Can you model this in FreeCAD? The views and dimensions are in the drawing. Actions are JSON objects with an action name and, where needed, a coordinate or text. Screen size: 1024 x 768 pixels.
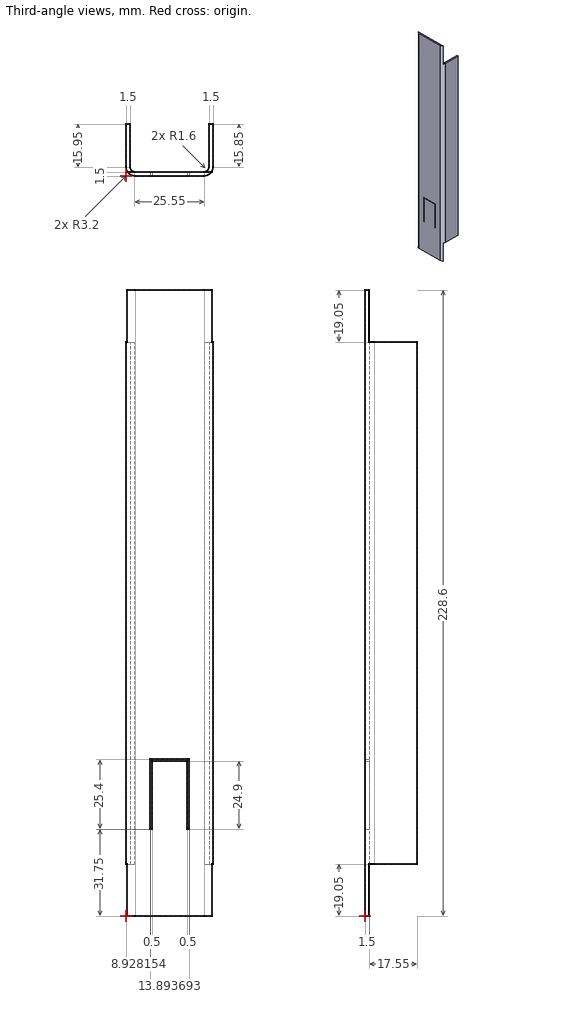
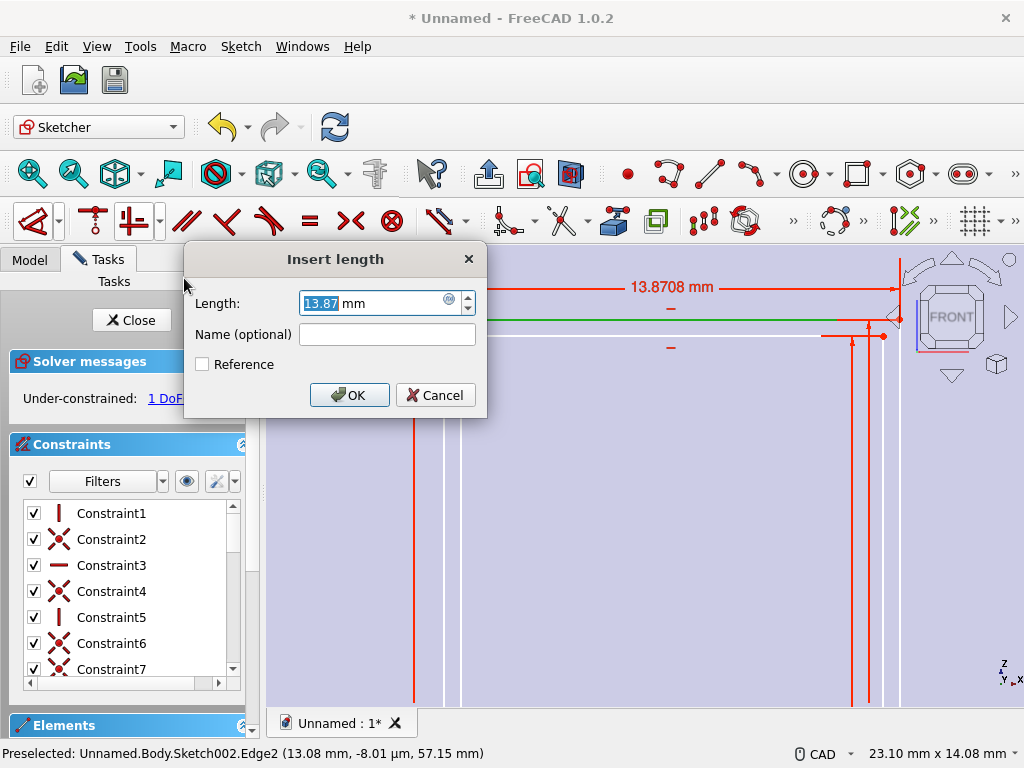
{"action": "type", "text": "13.893693"}
{"action": "key", "text": "Return"}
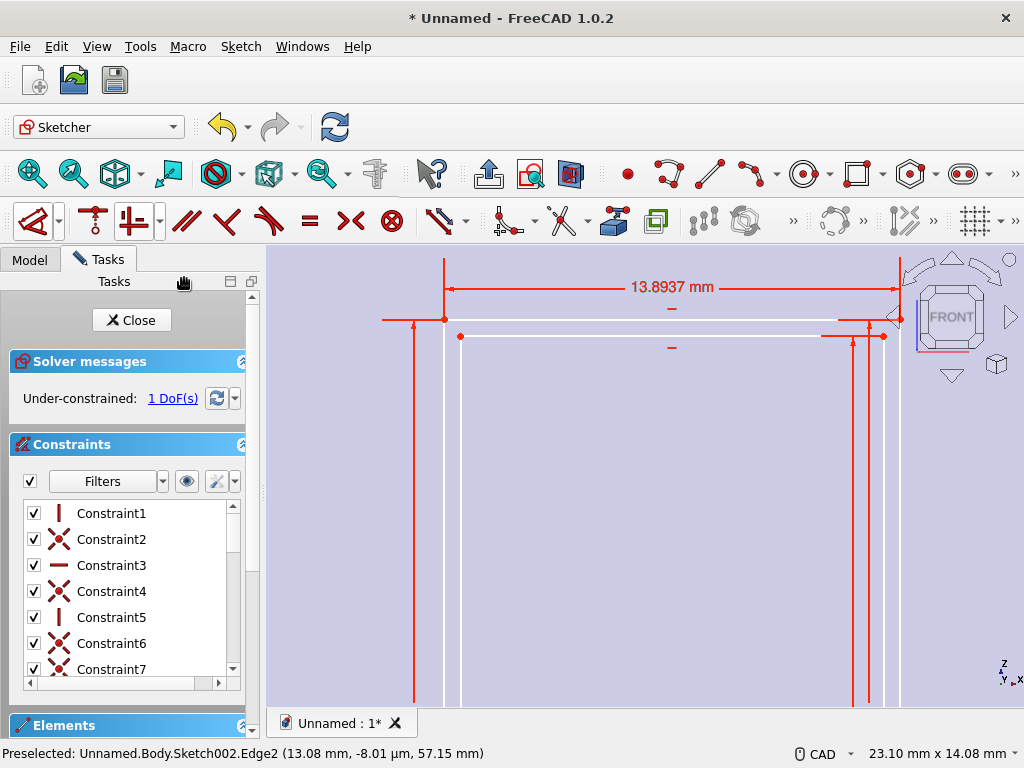
{"action": "scroll", "coordinate": [586, 321], "scroll_direction": "down", "scroll_amount": 9}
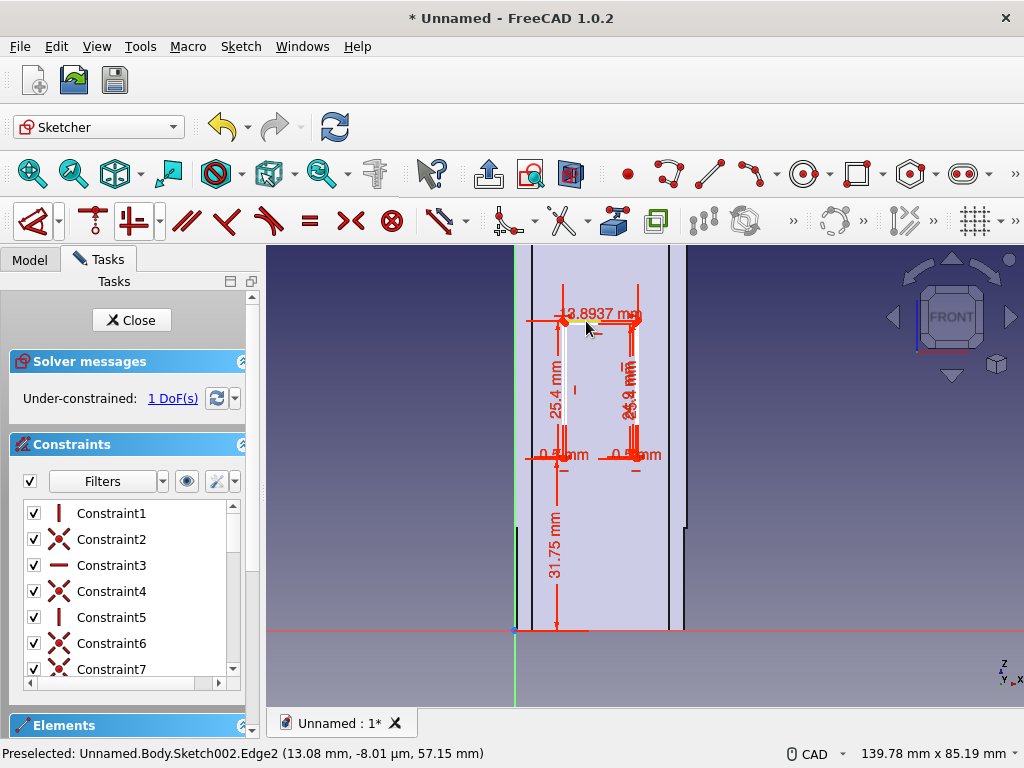
{"action": "scroll", "coordinate": [563, 459], "scroll_direction": "up", "scroll_amount": 8}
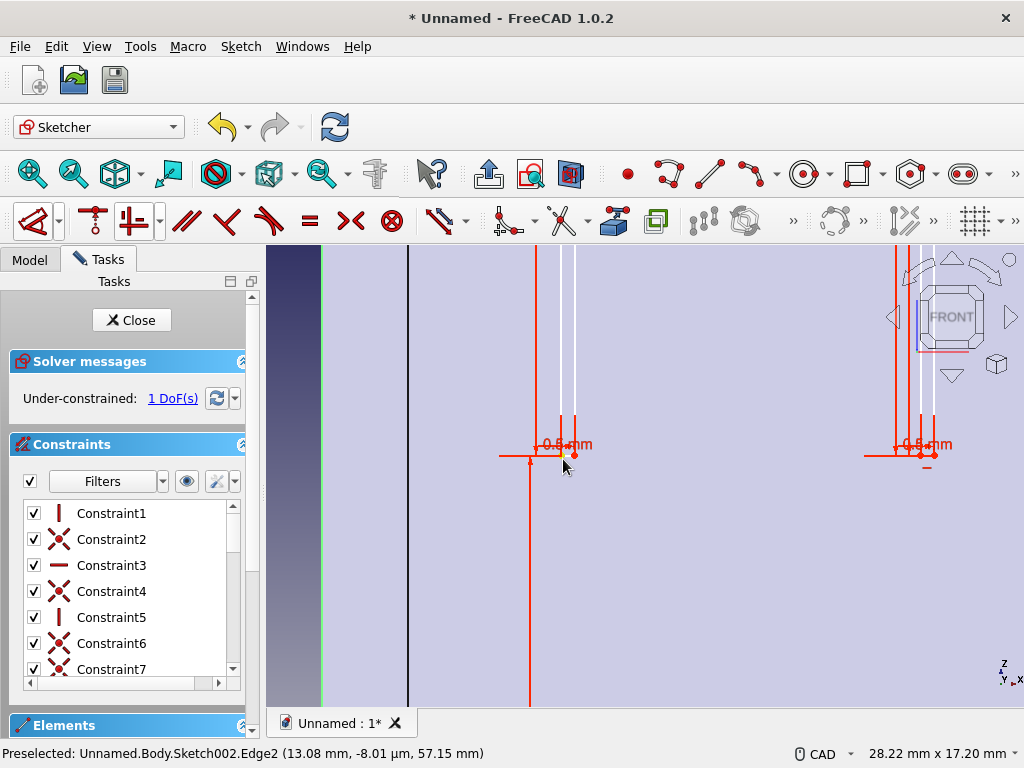
{"action": "left_click", "coordinate": [561, 456]}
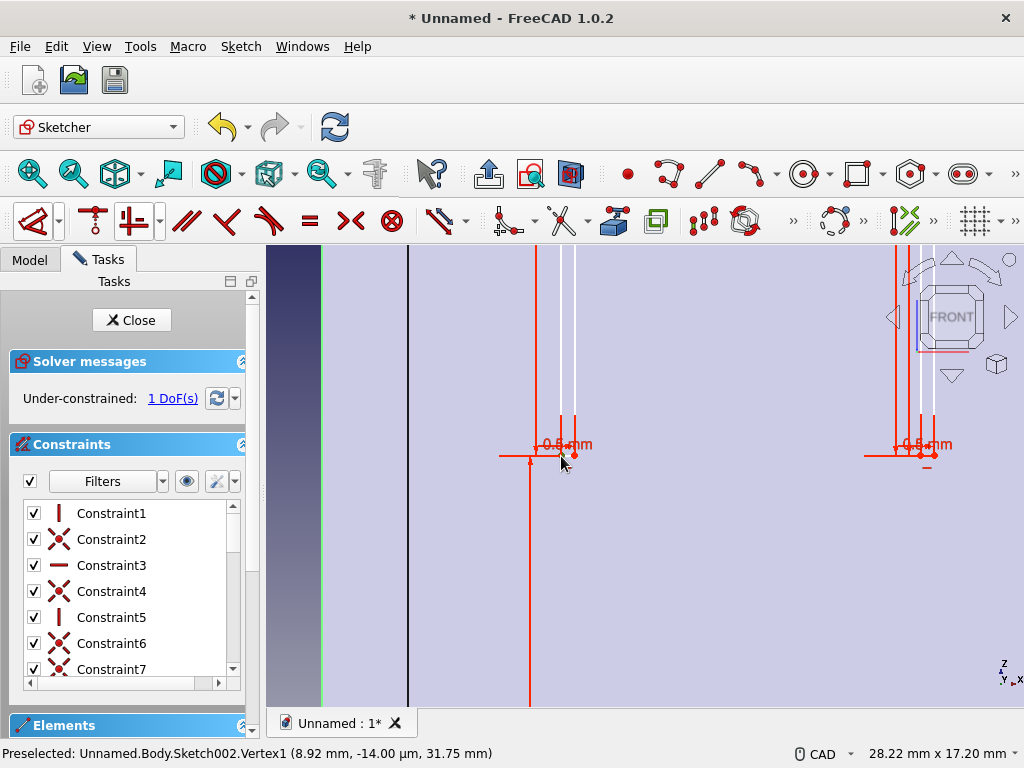
{"action": "left_click", "coordinate": [58, 222]}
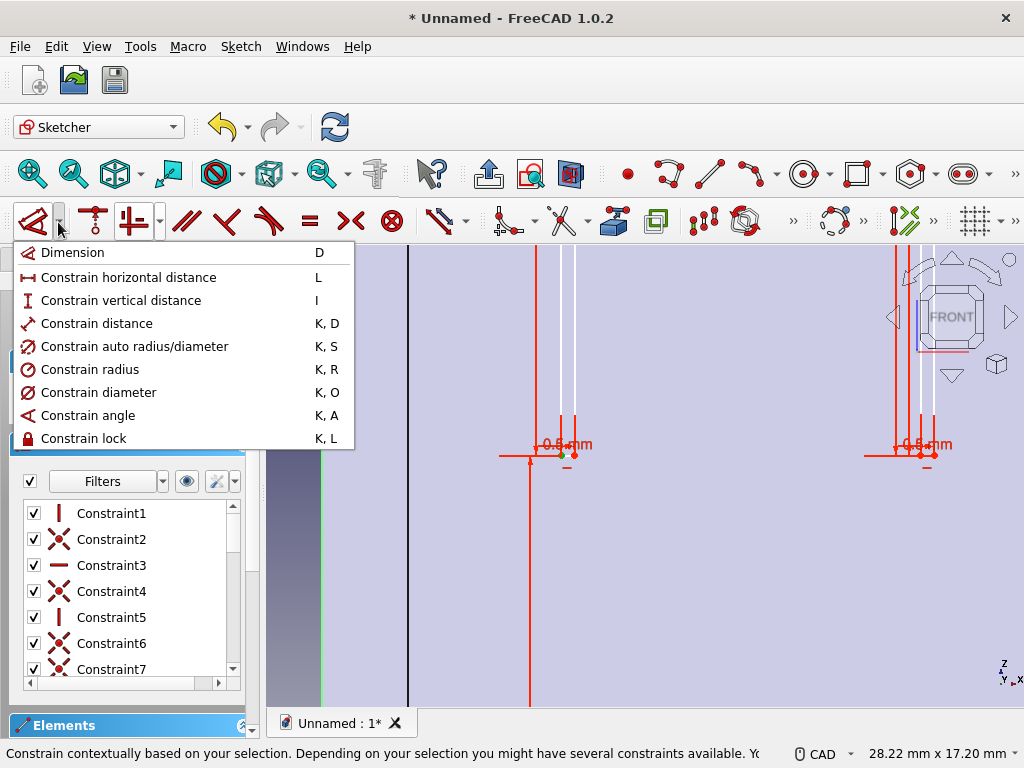
{"action": "left_click", "coordinate": [184, 278]}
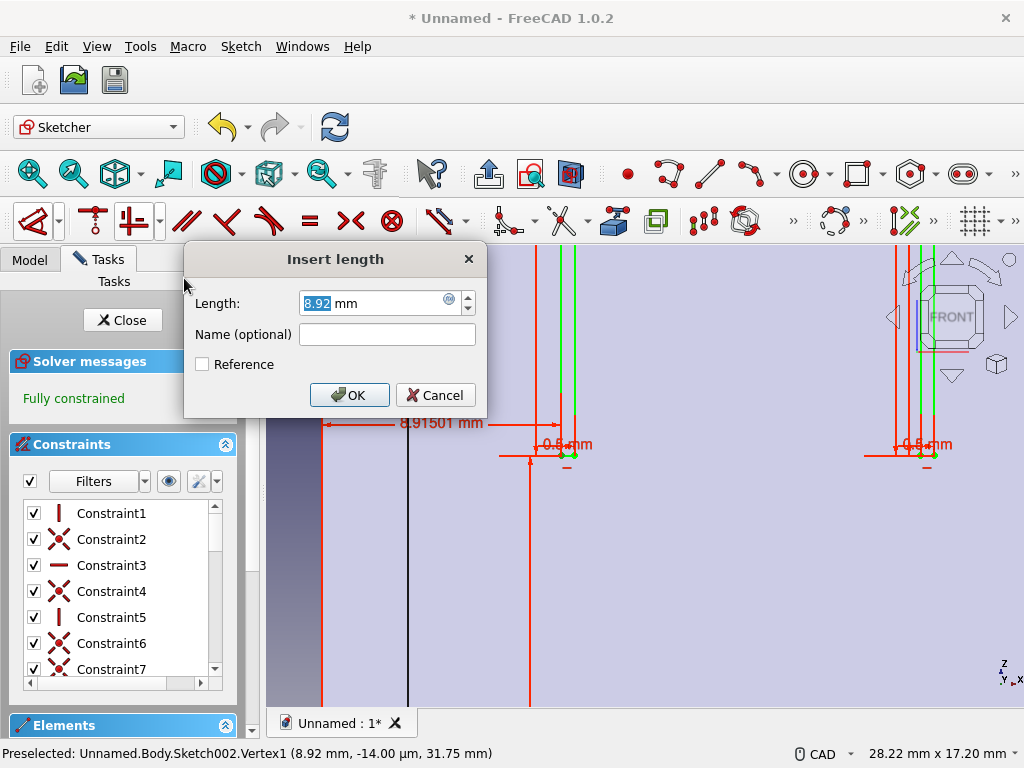
{"action": "type", "text": "8.928154"}
{"action": "key", "text": "Return"}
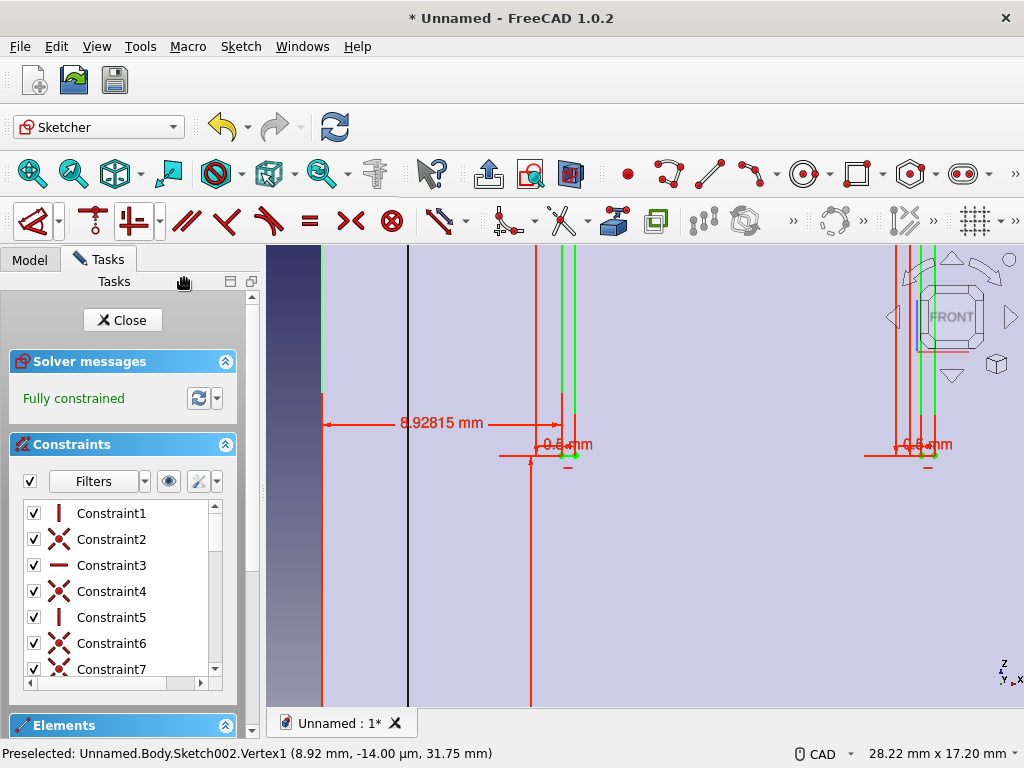
{"action": "left_click", "coordinate": [123, 320]}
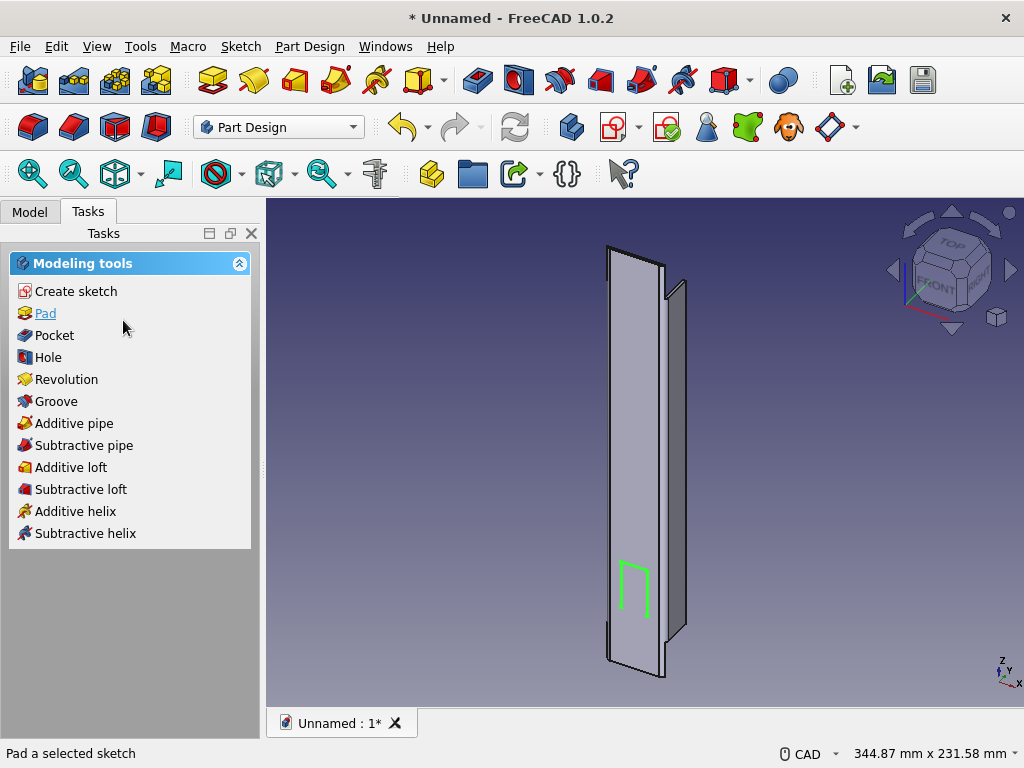
{"action": "left_click", "coordinate": [478, 80]}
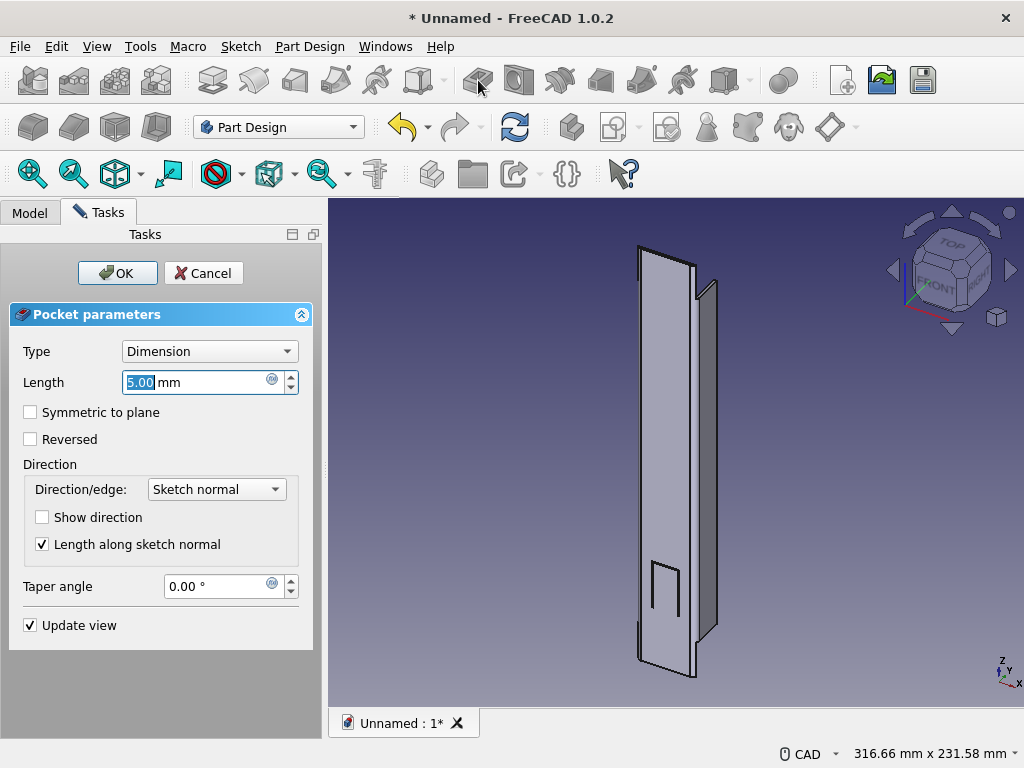
{"action": "left_click", "coordinate": [210, 352]}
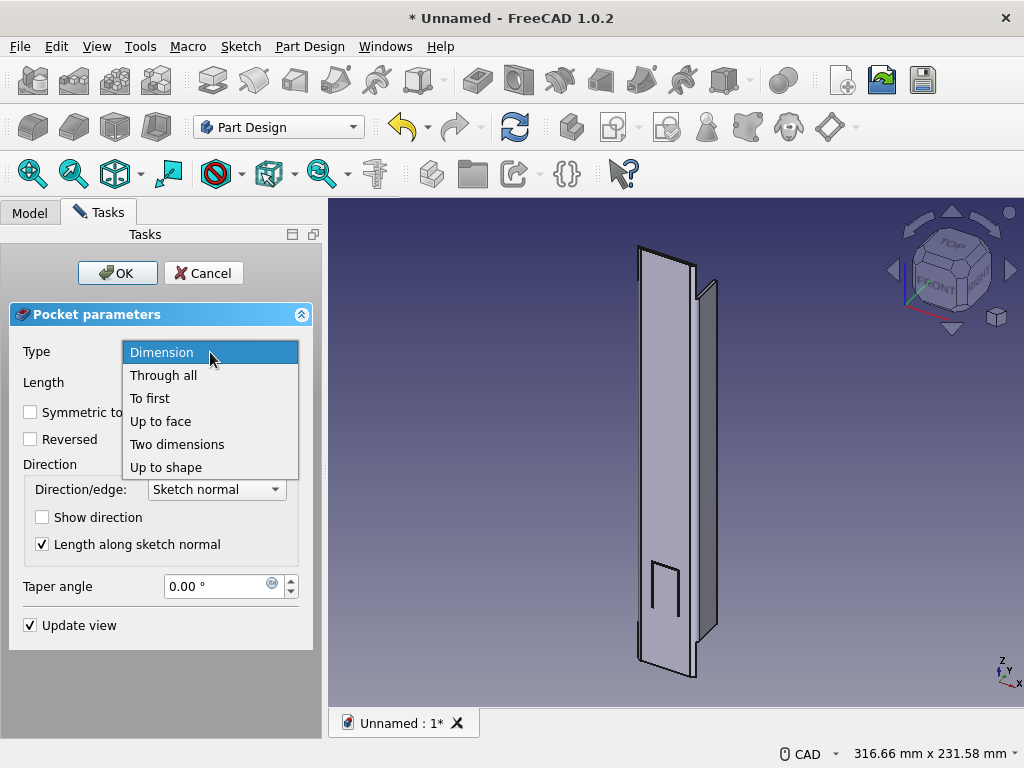
{"action": "left_click", "coordinate": [208, 376]}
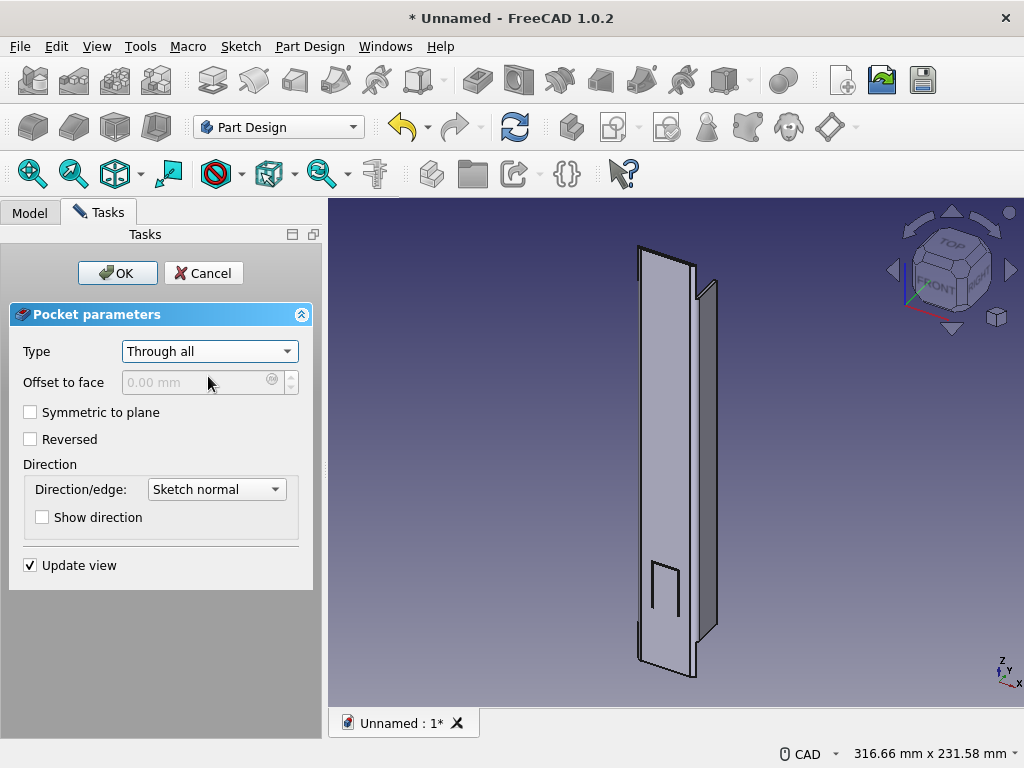
{"action": "left_click", "coordinate": [118, 273]}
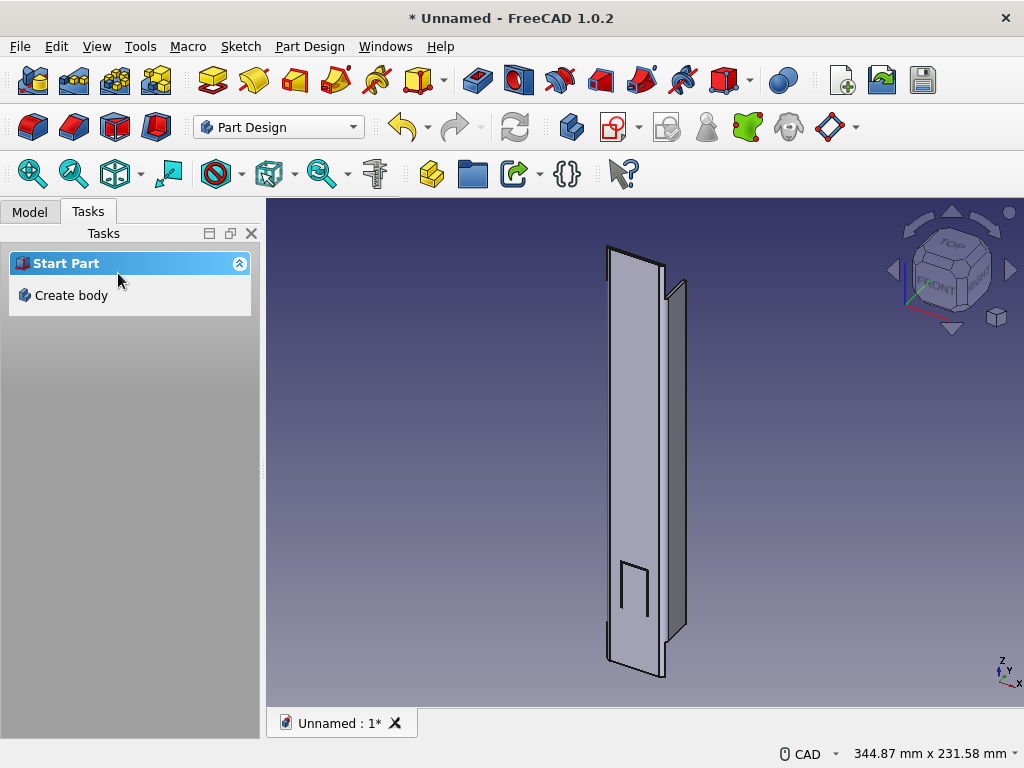
{"action": "key", "text": "0"}